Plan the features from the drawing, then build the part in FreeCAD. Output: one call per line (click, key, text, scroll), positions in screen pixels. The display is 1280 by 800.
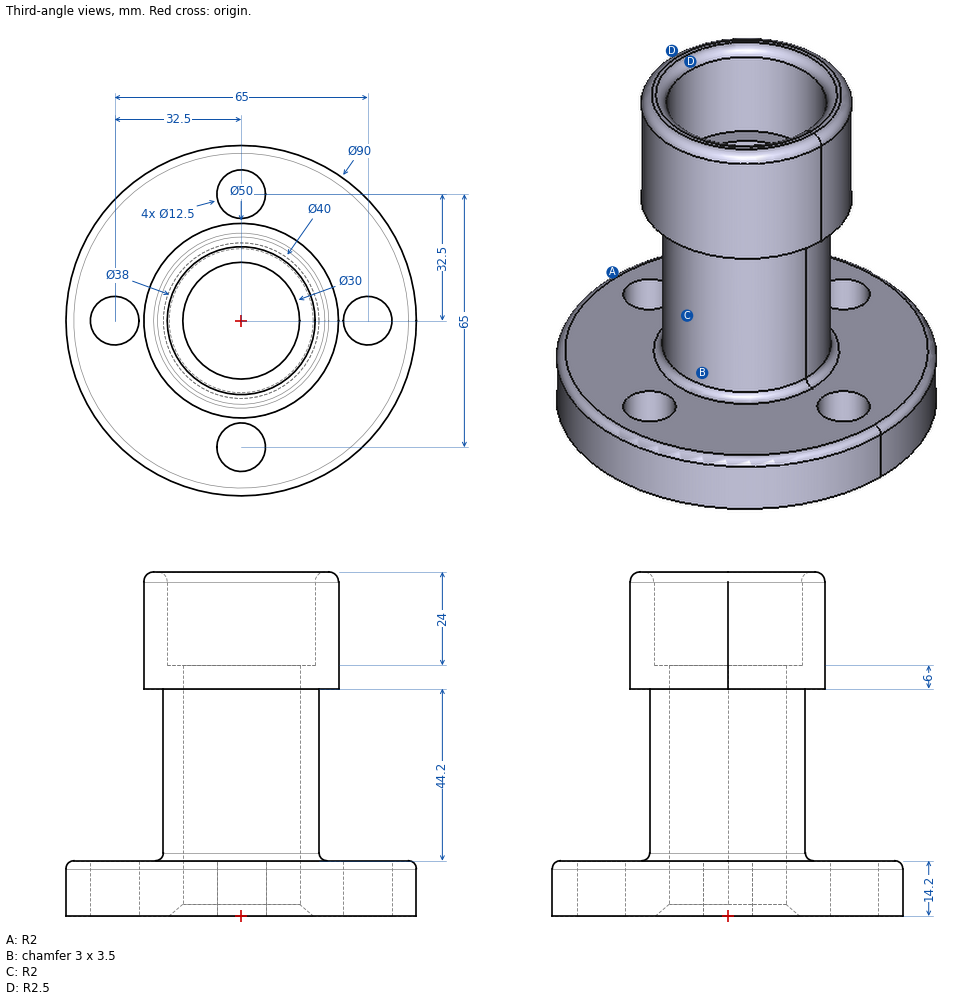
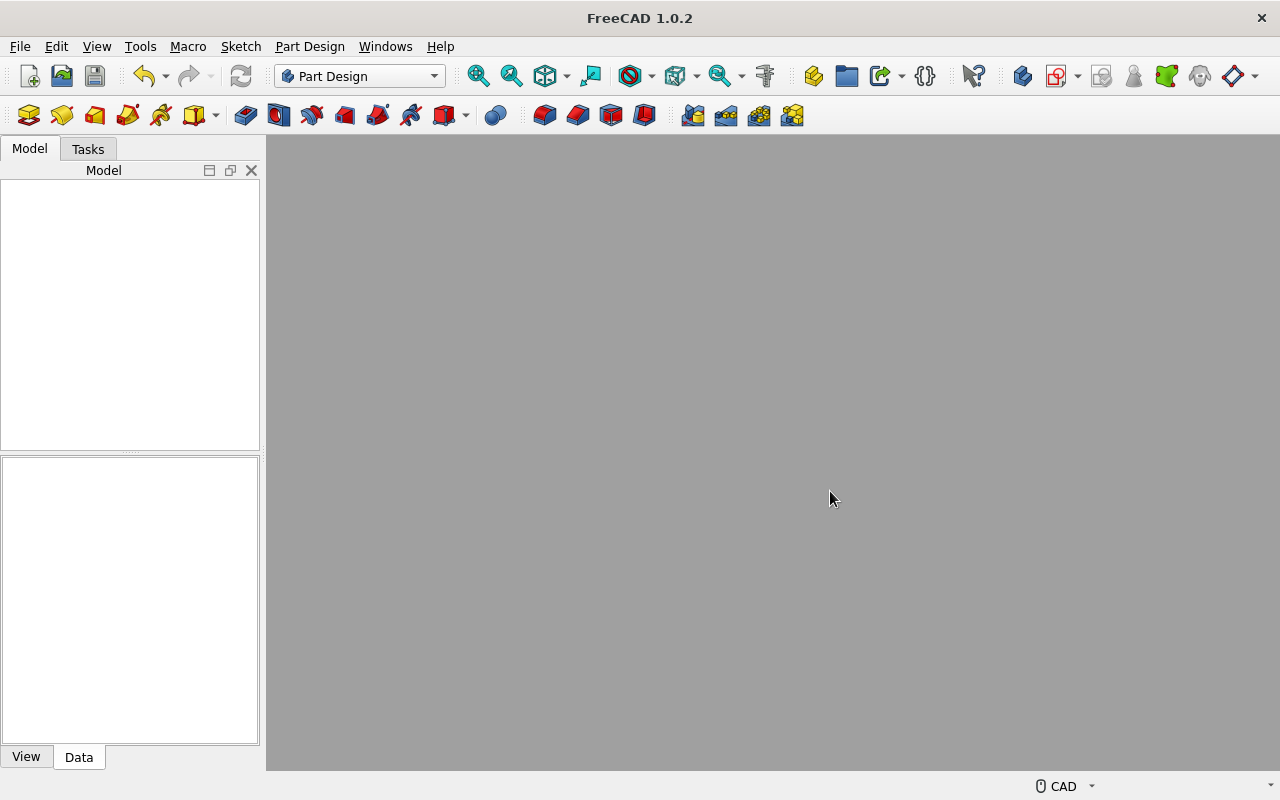
click(29, 76)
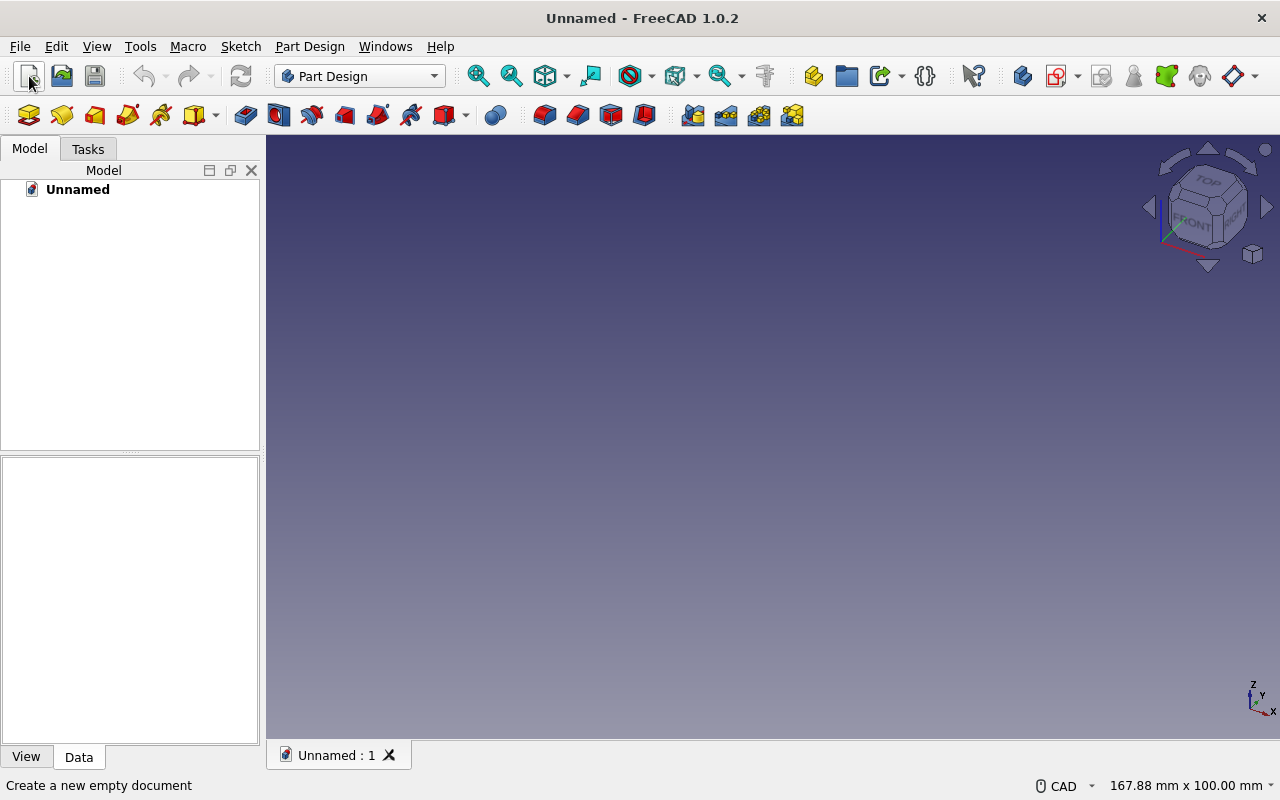
click(1056, 76)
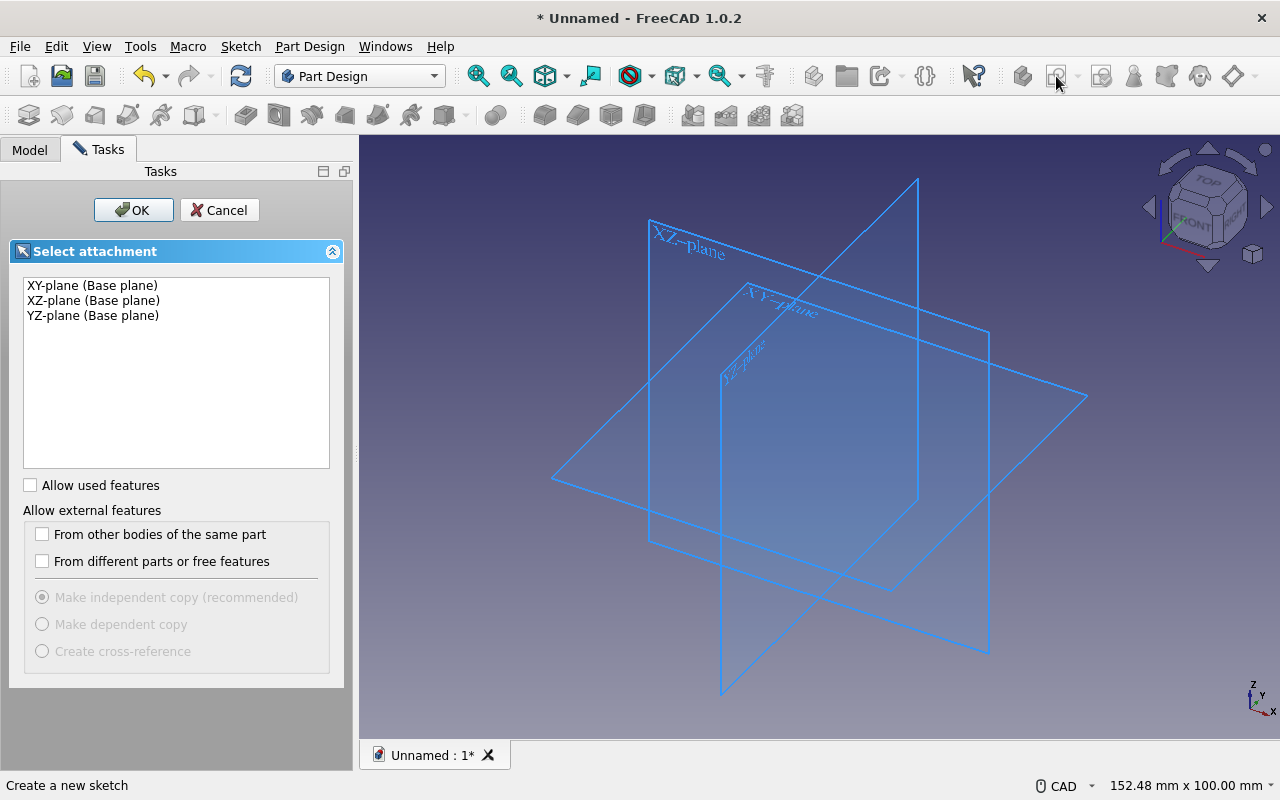
click(84, 286)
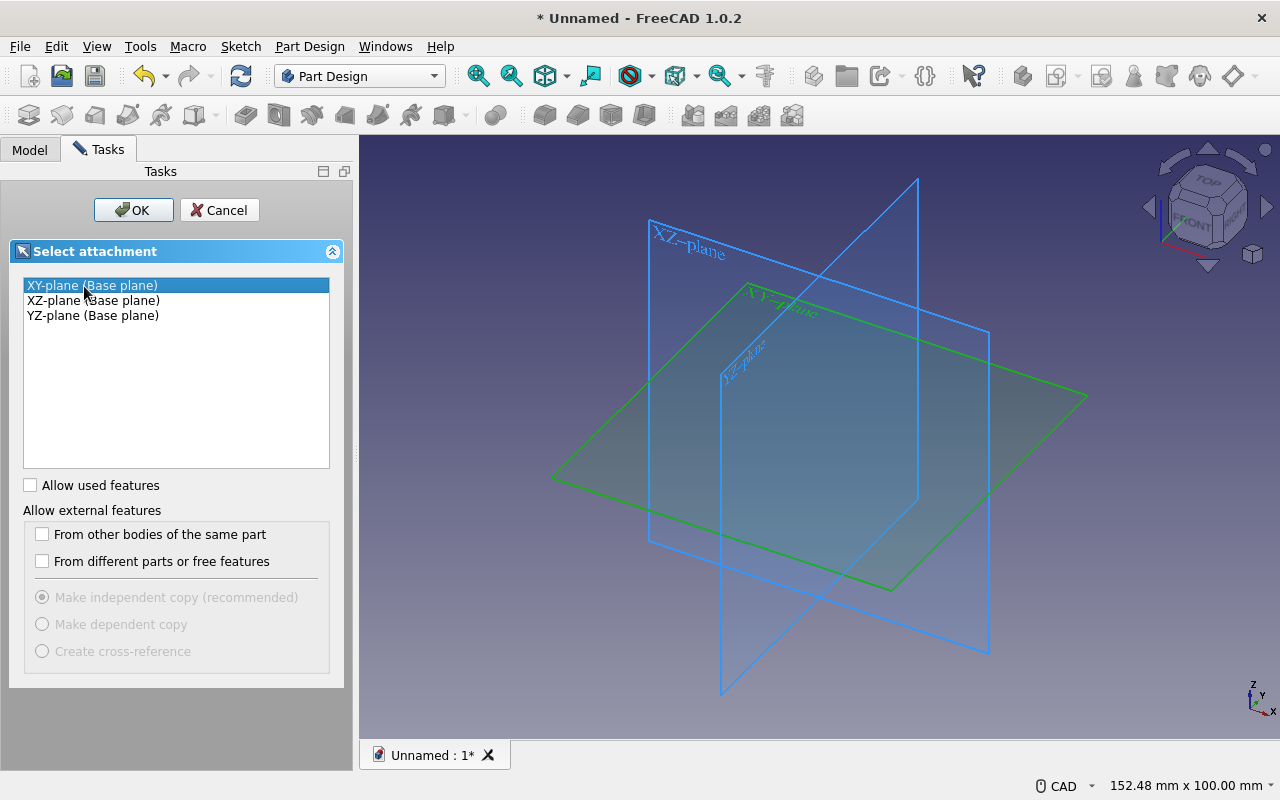
click(134, 210)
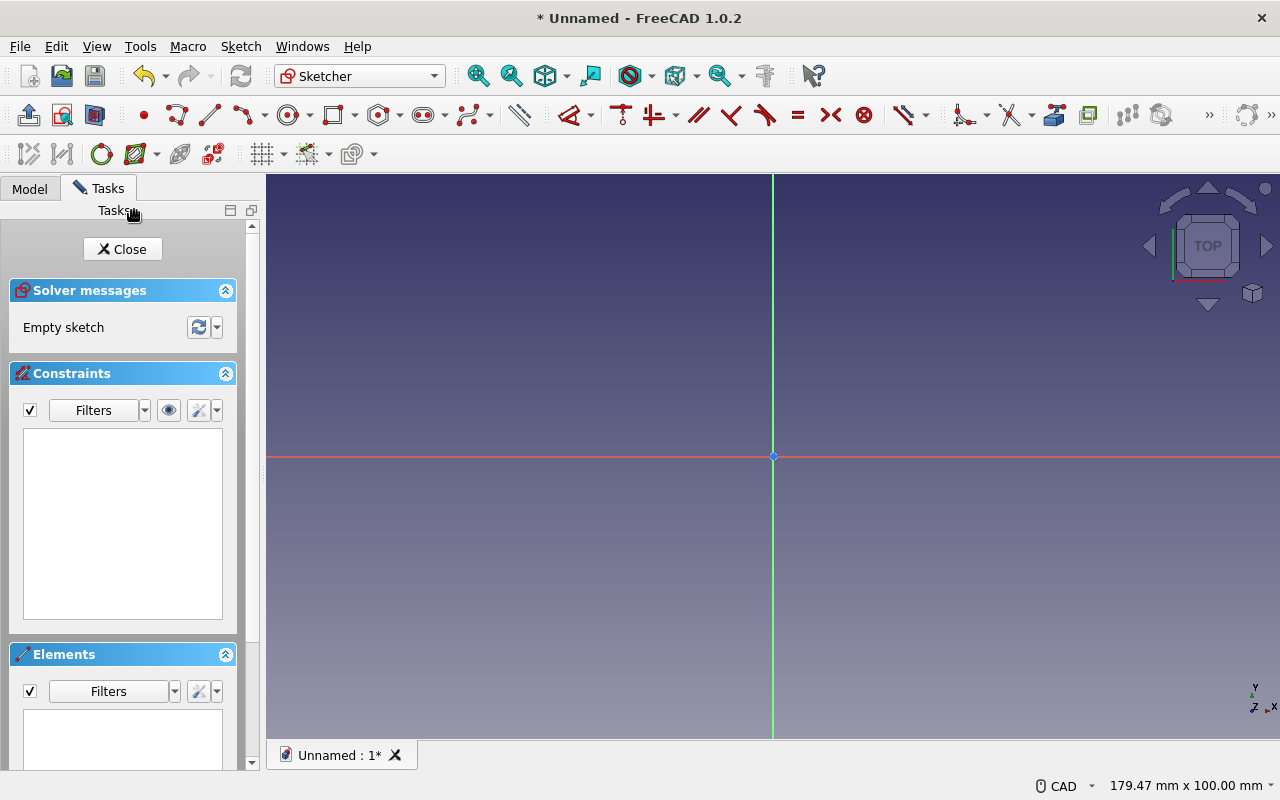
scroll(565, 457, down, 2)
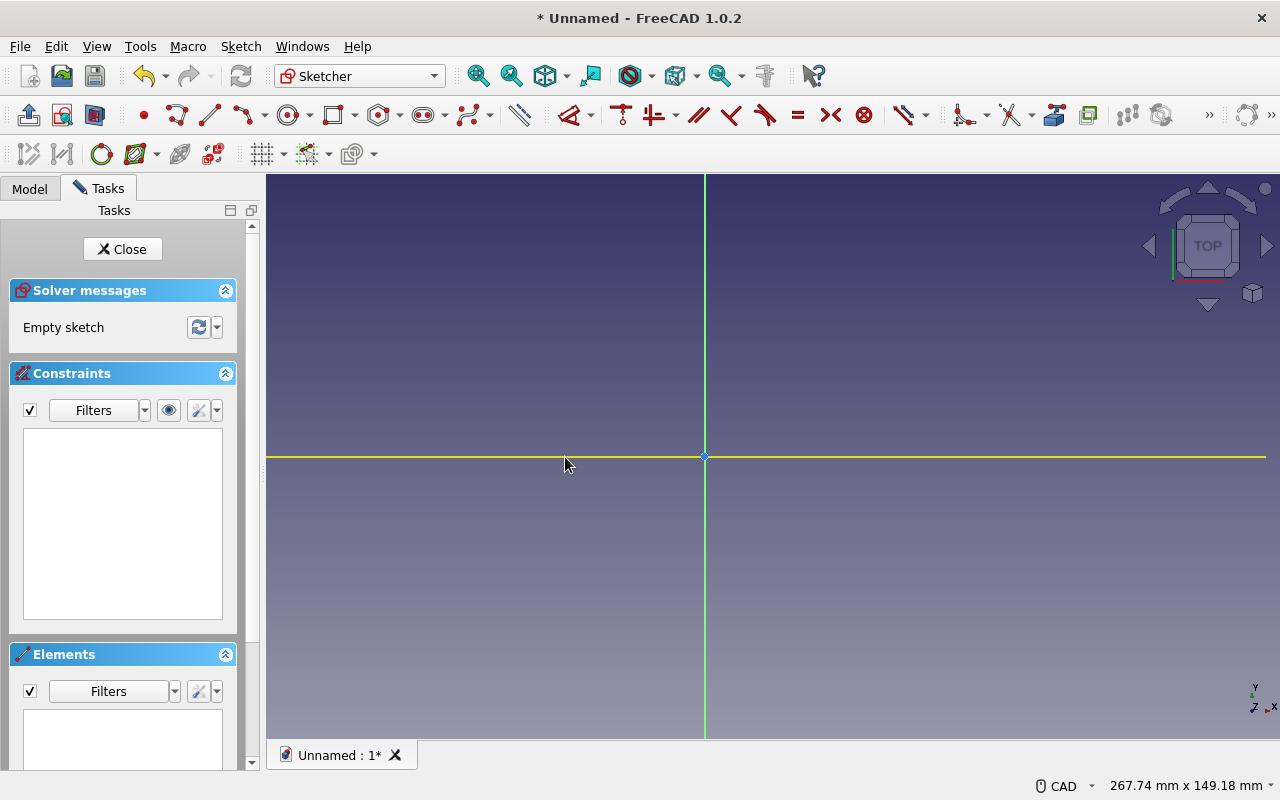
click(288, 116)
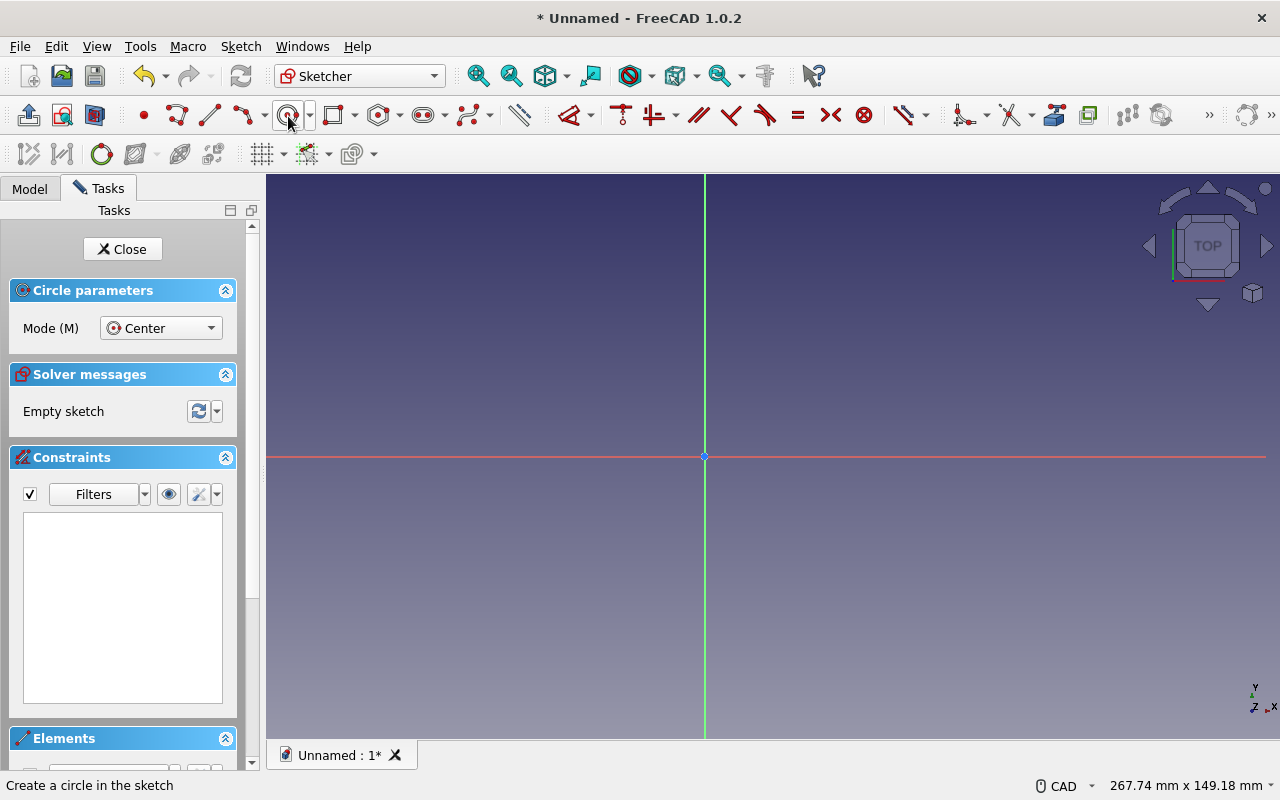
click(705, 457)
move(825, 336)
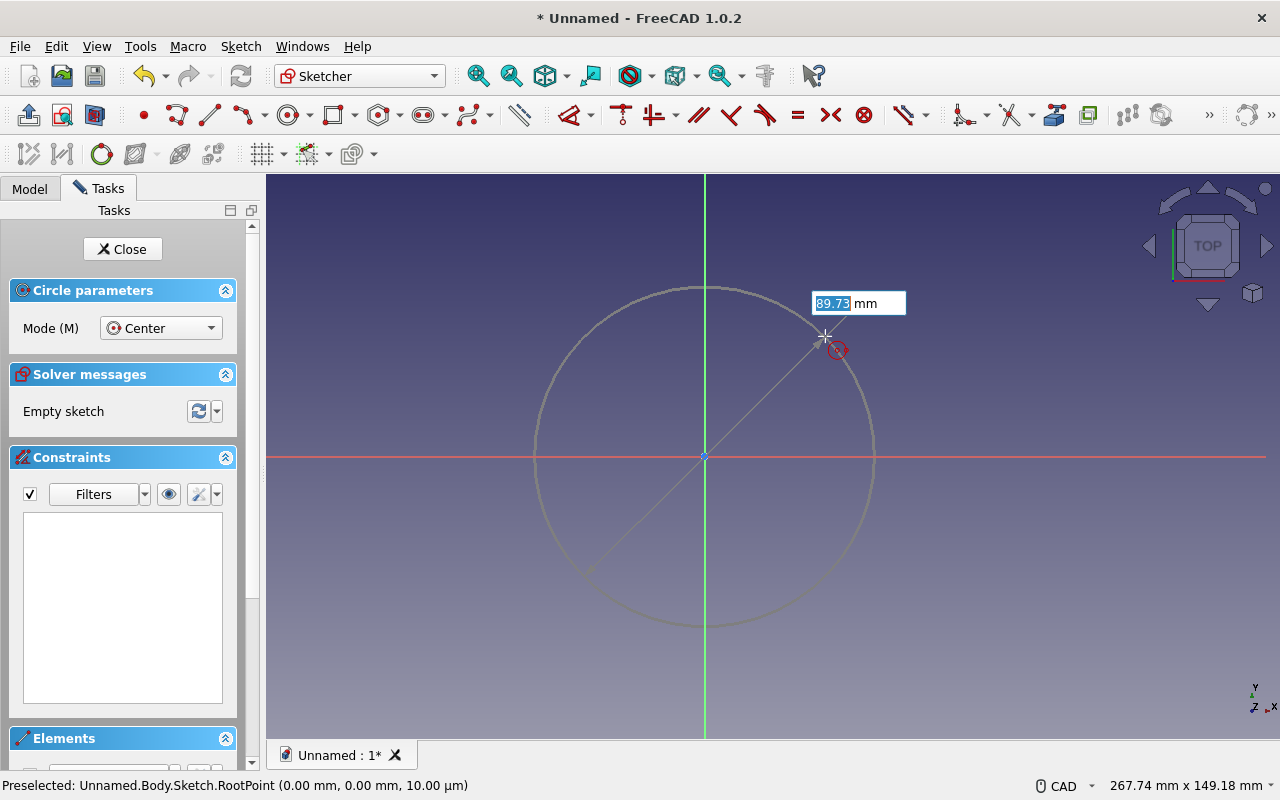
text(90)
key(Return)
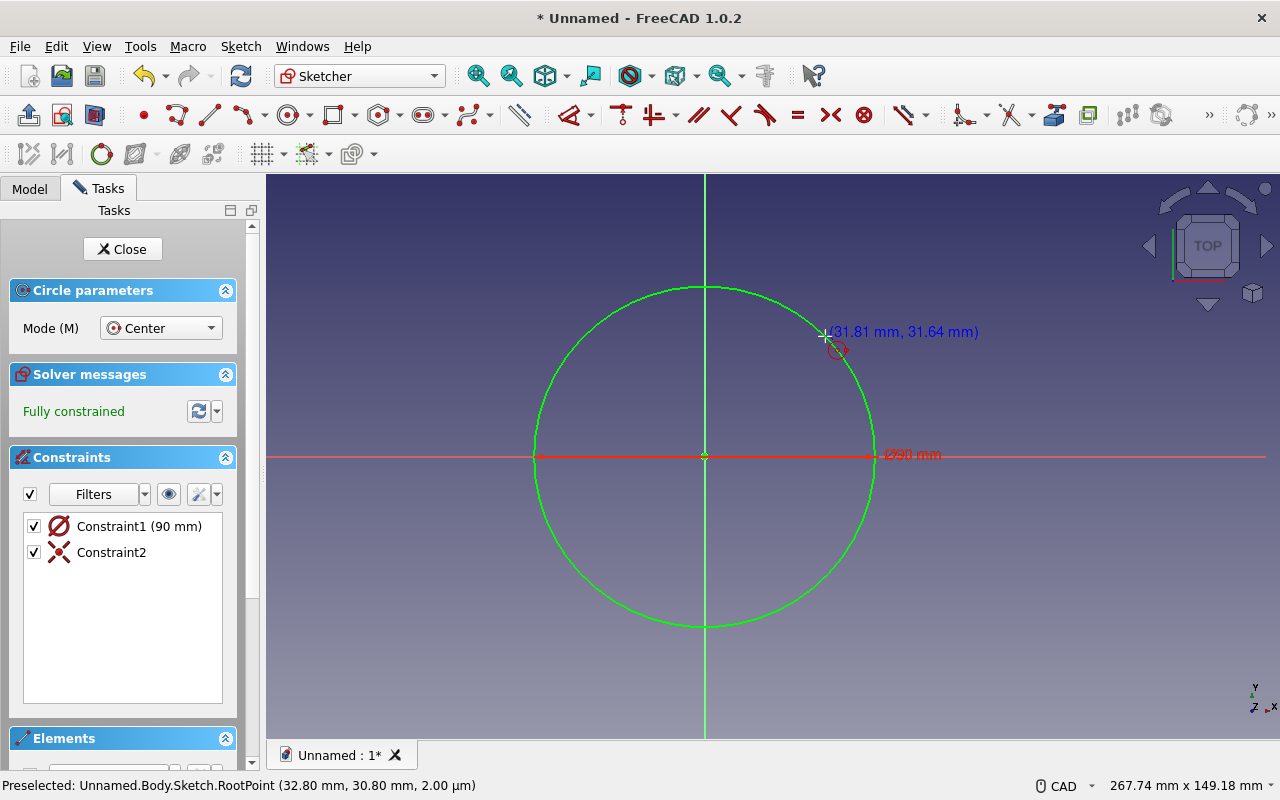
click(705, 457)
move(745, 417)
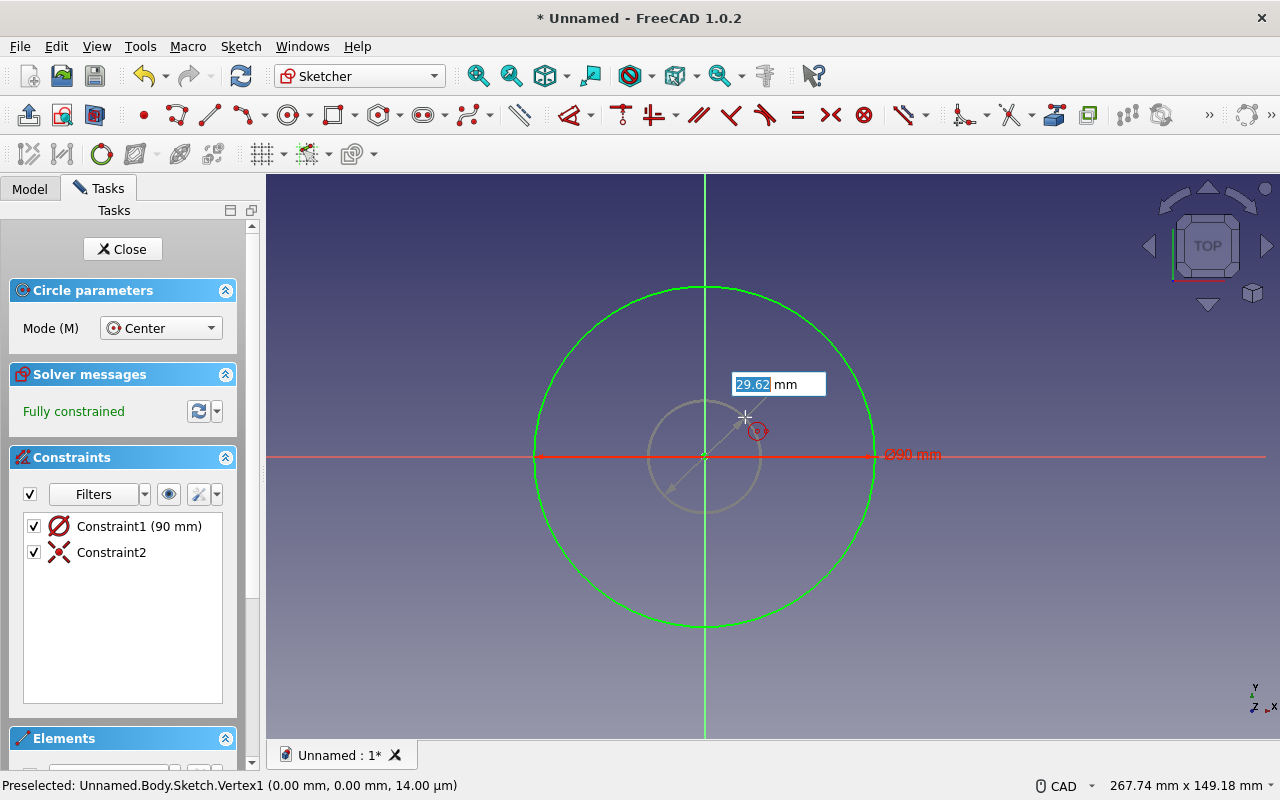
text(30)
key(Return)
key(Escape)